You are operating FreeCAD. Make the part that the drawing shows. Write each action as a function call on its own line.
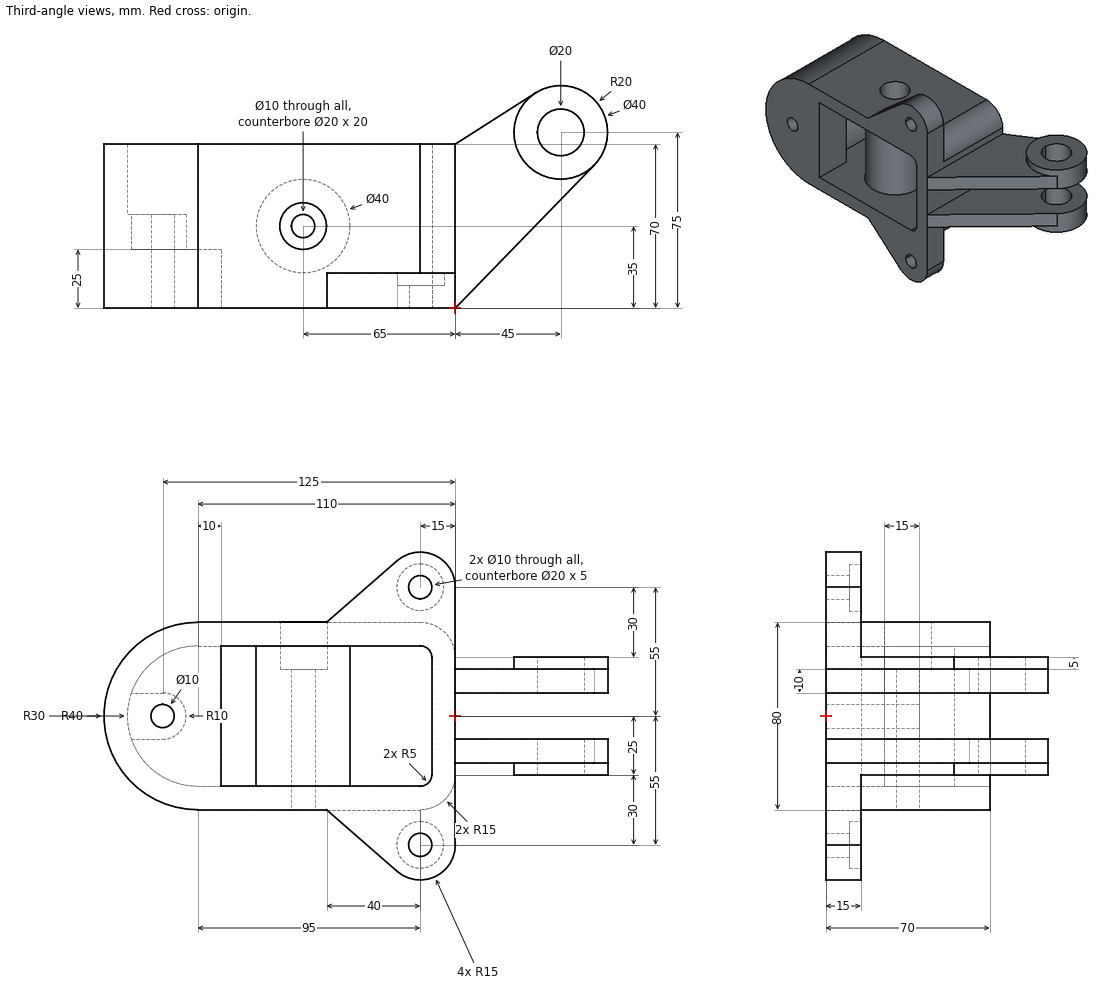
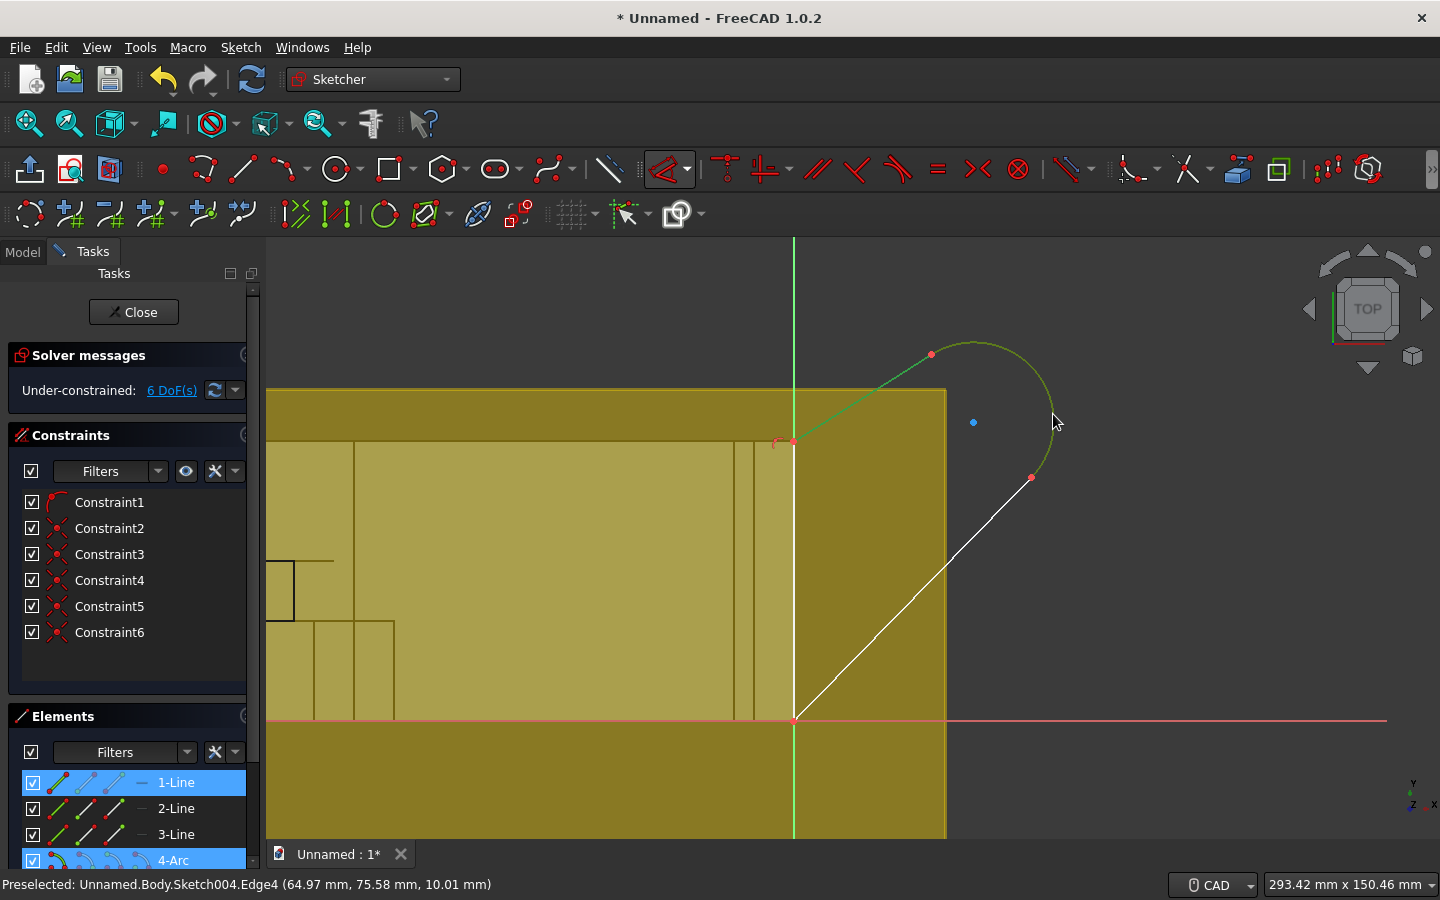
key(t)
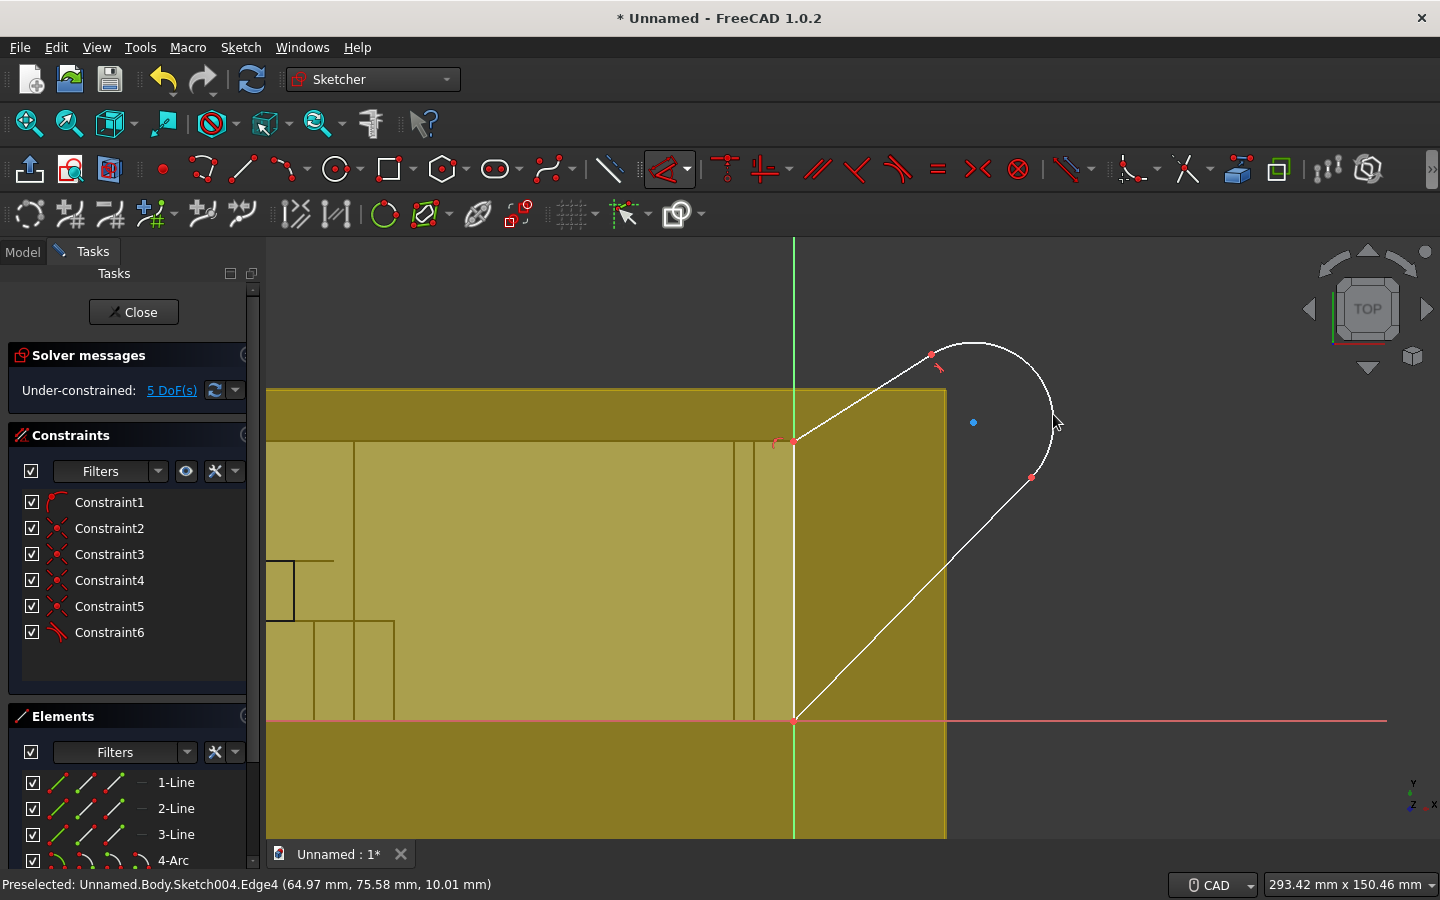
click(865, 648)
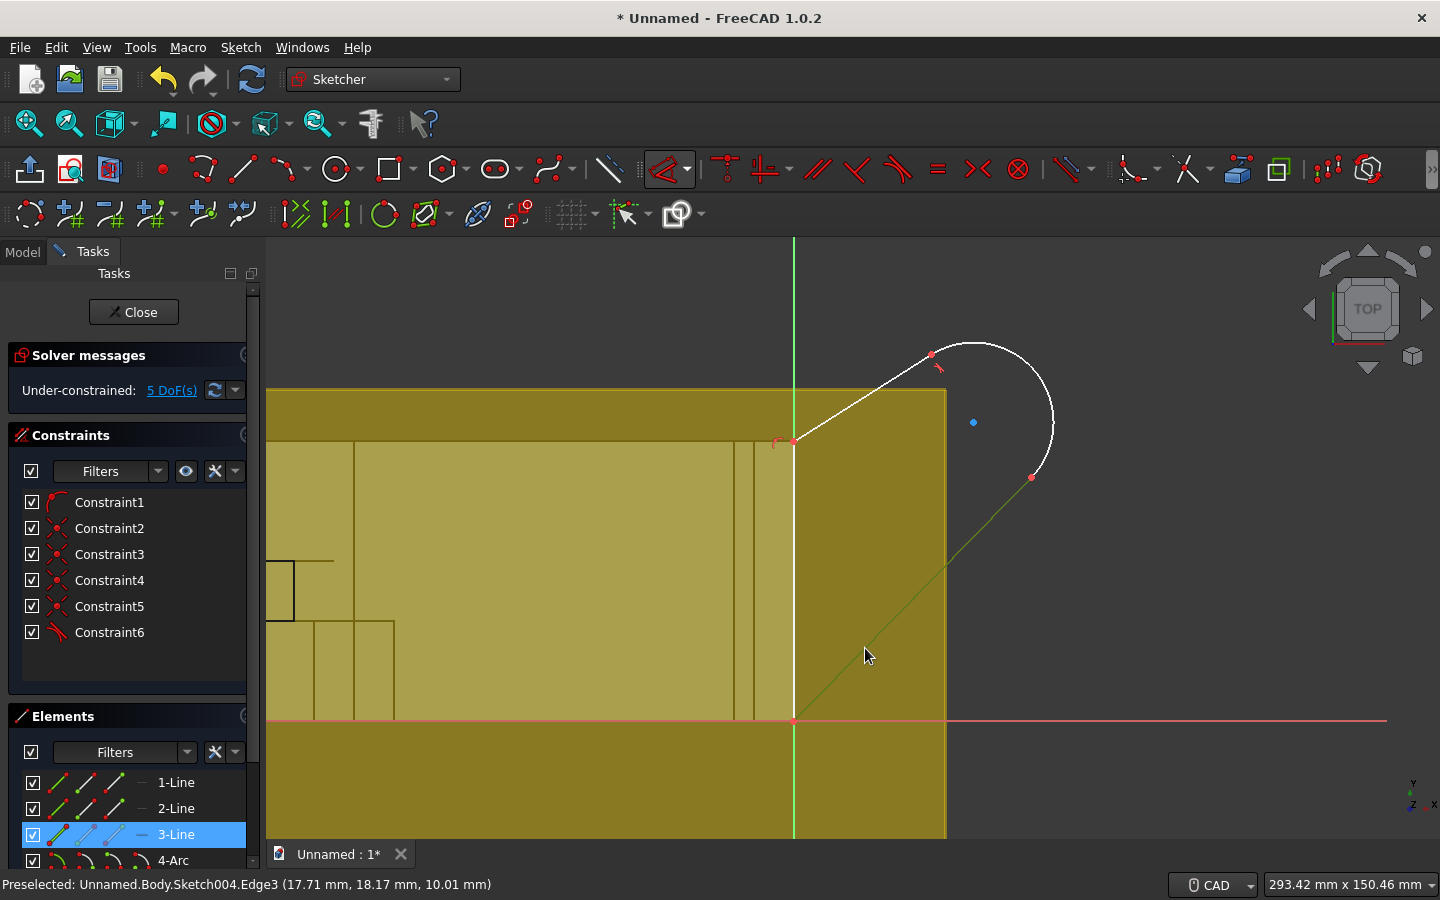
click(1053, 414)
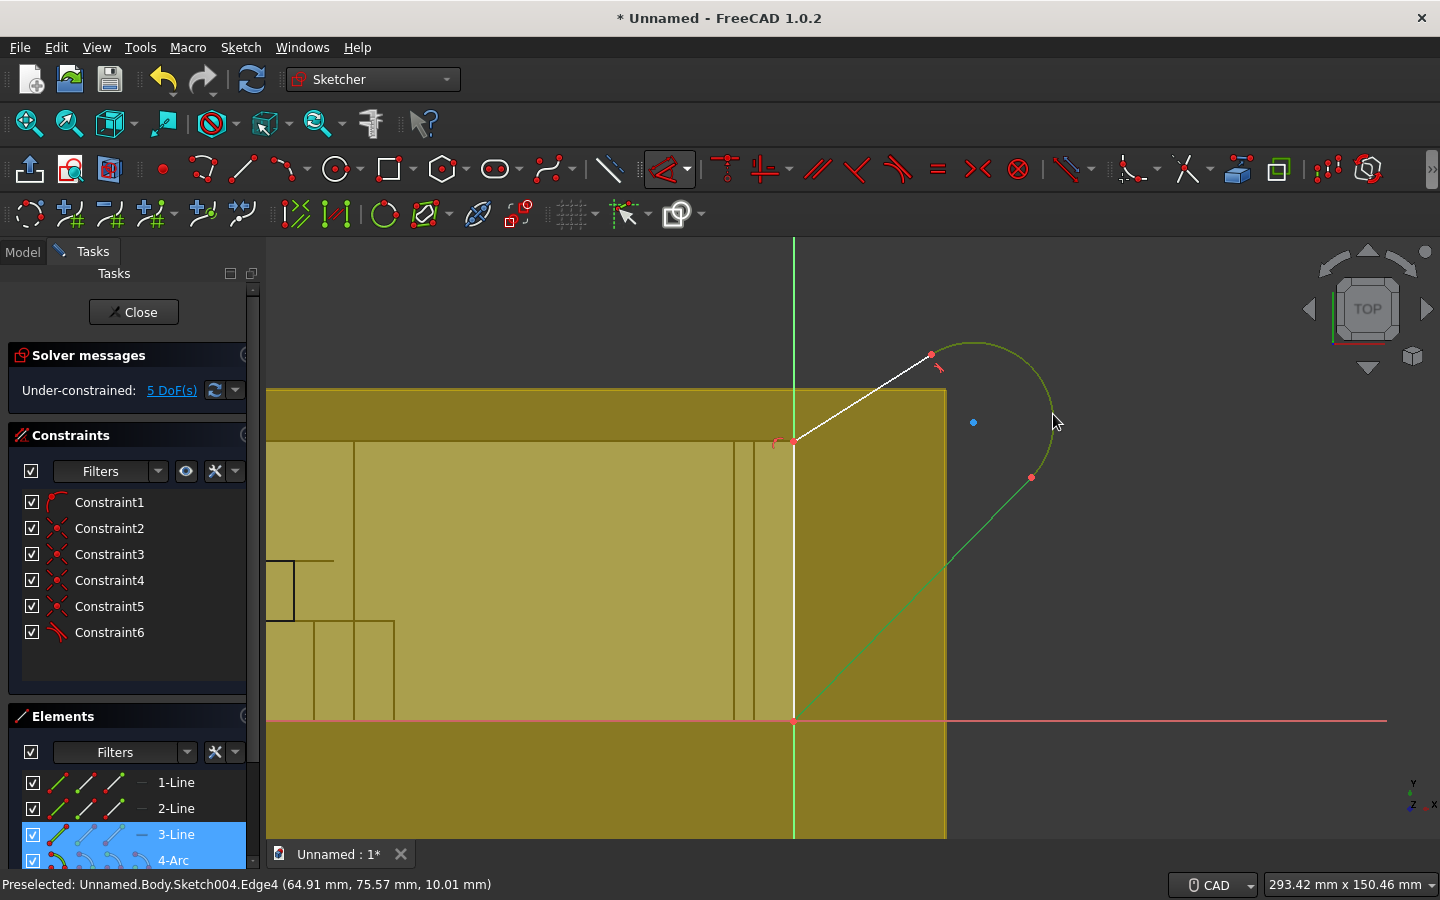
key(t)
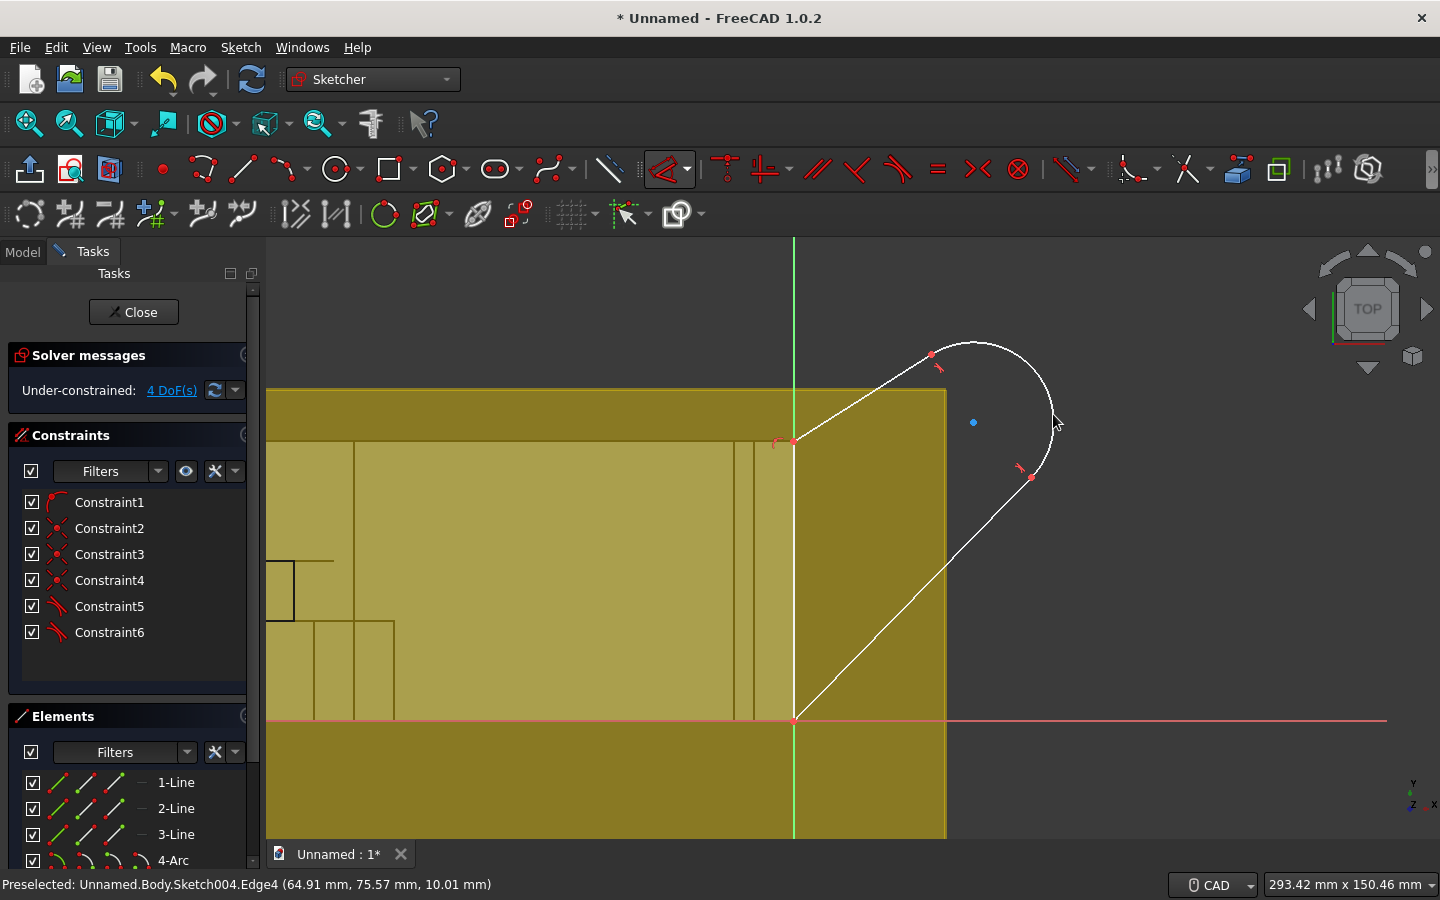
click(1053, 414)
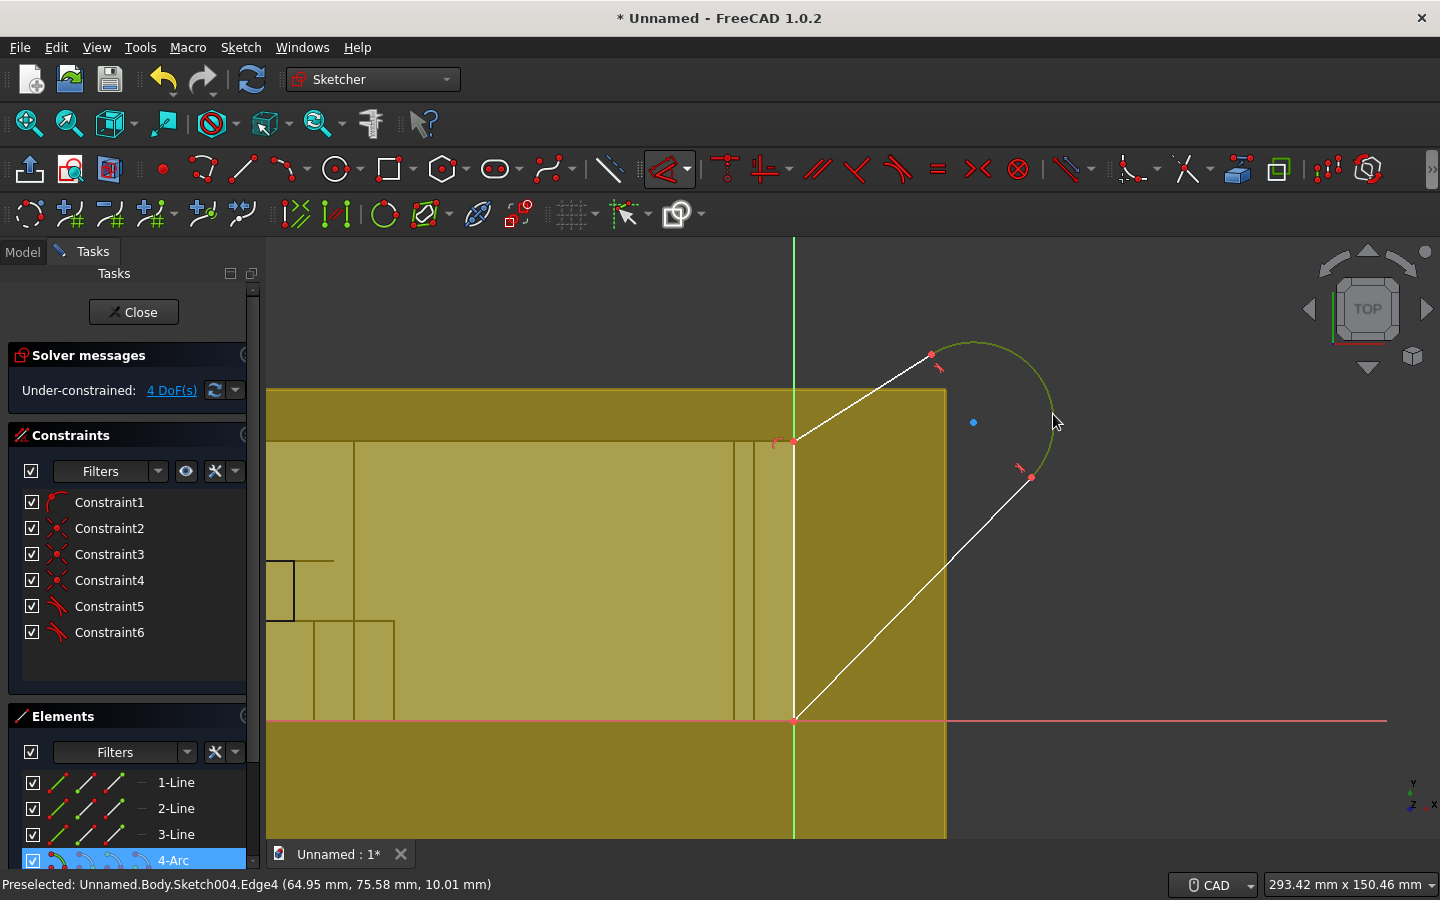
click(690, 170)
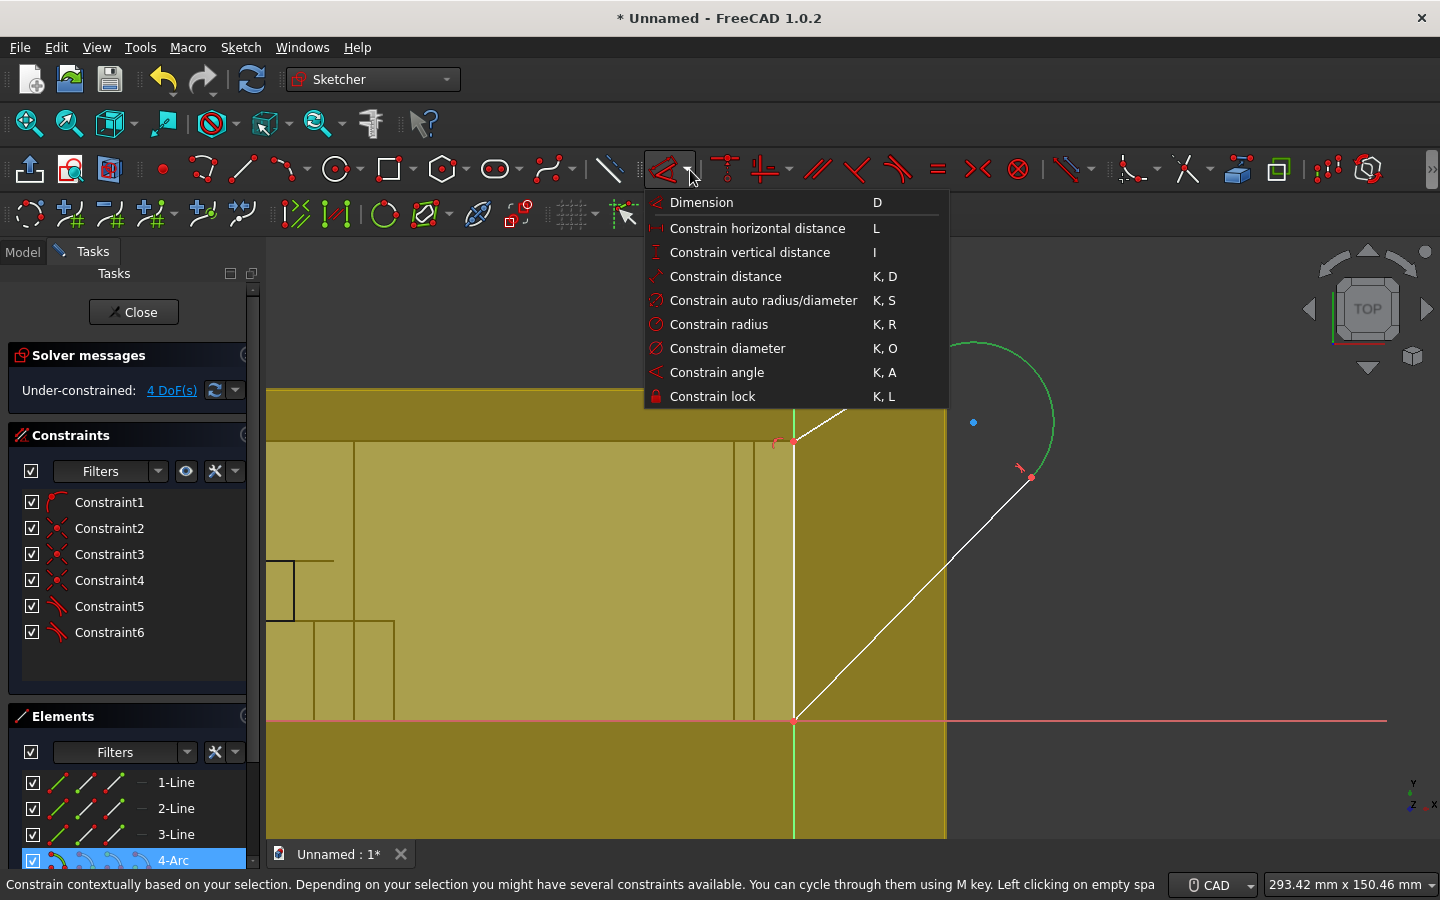
click(797, 324)